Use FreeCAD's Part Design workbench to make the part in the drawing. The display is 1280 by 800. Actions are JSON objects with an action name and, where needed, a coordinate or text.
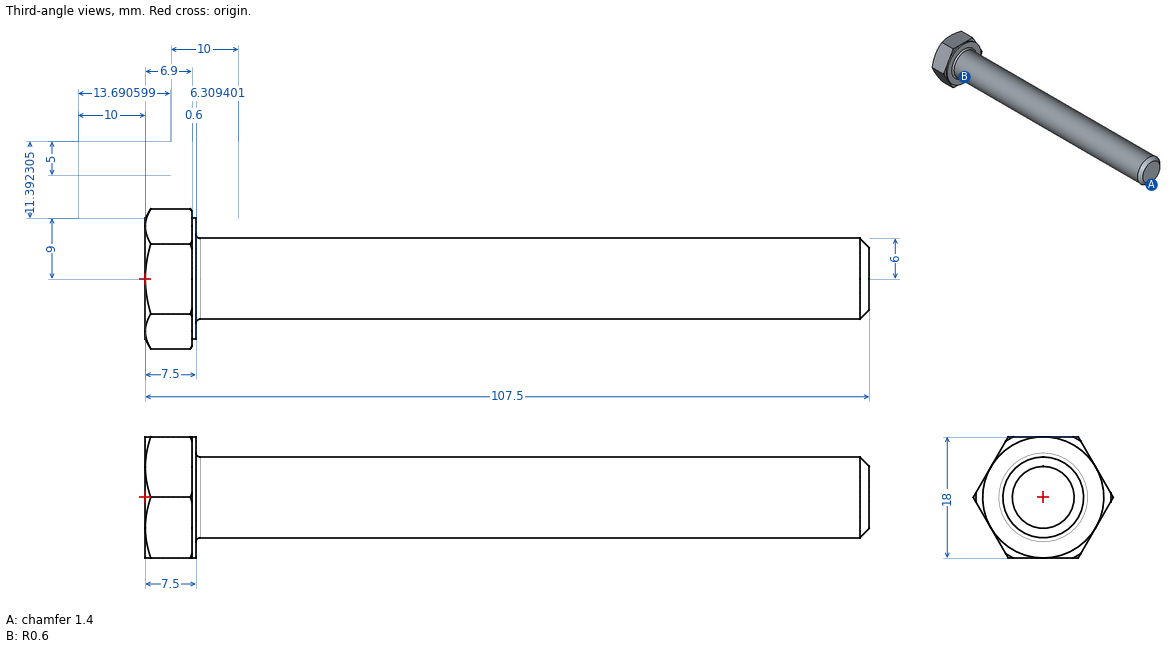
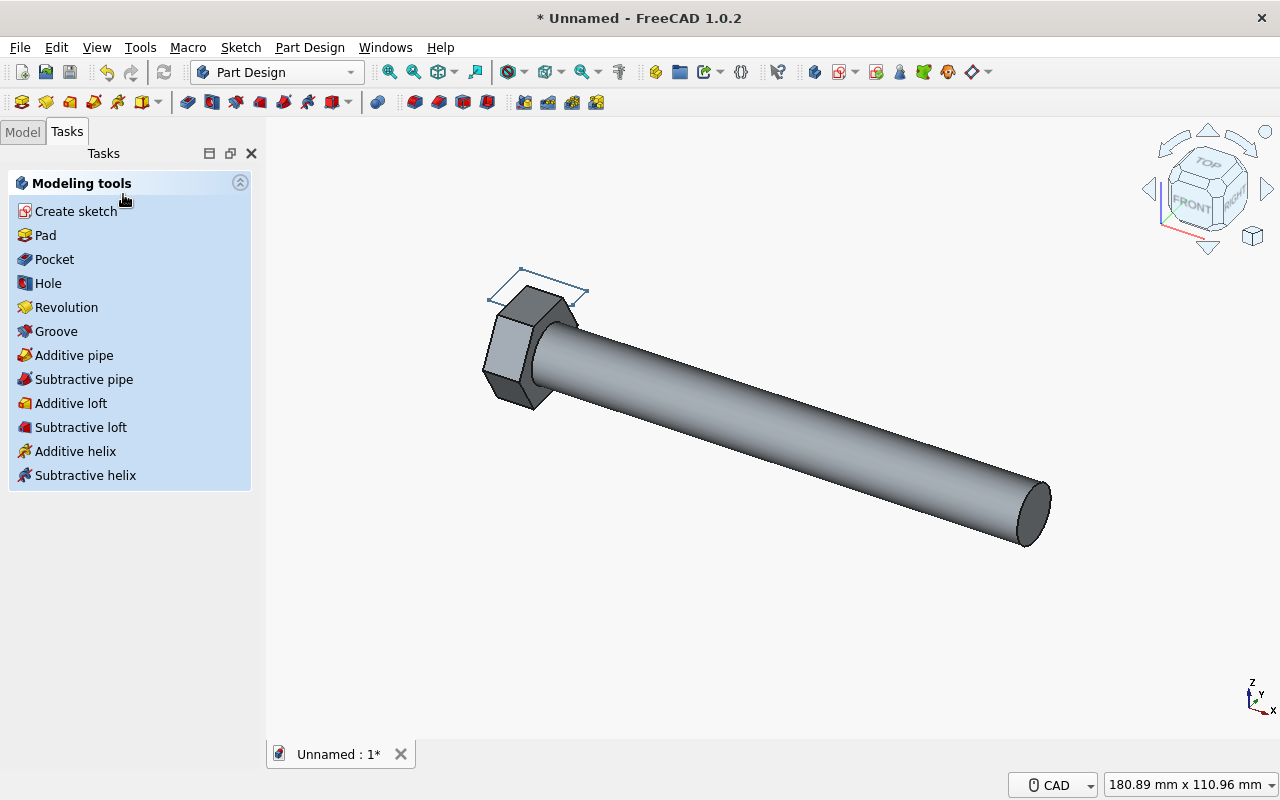
{"action": "left_click", "coordinate": [236, 102]}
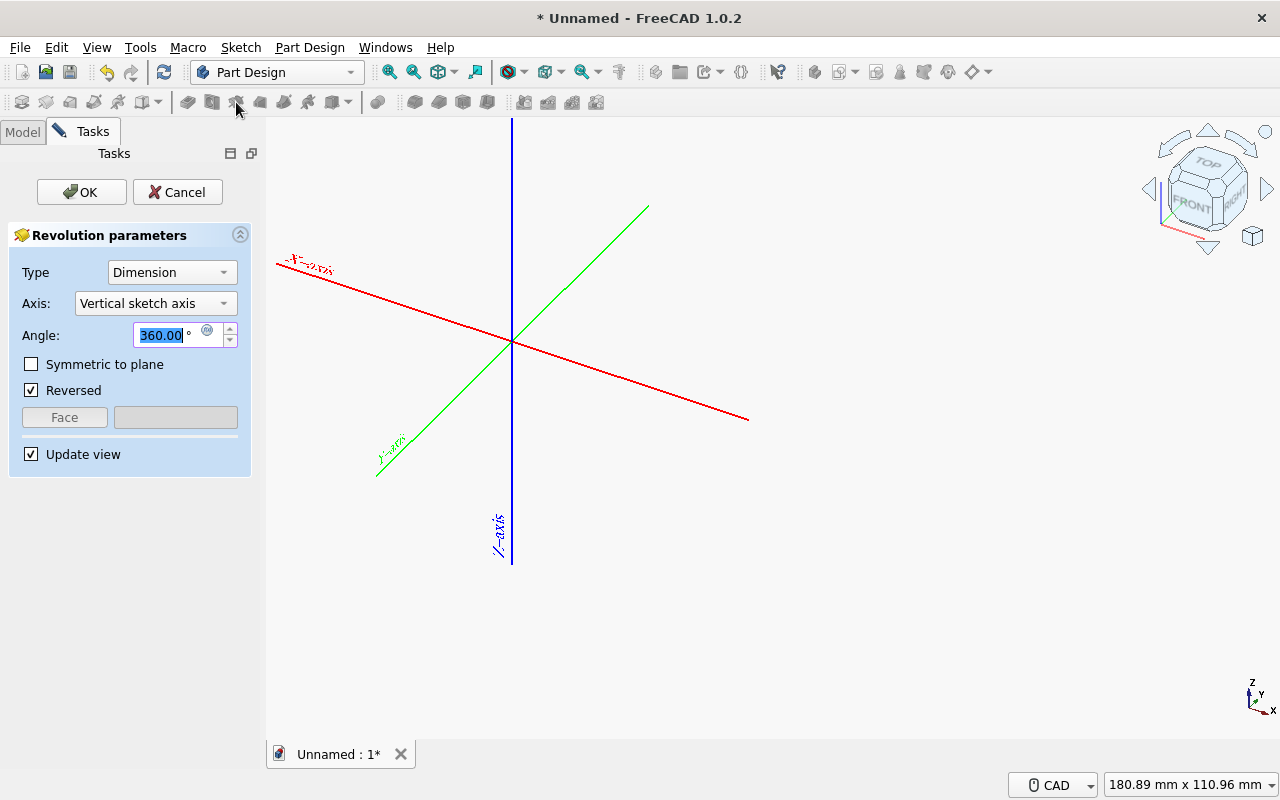
{"action": "left_click", "coordinate": [156, 304]}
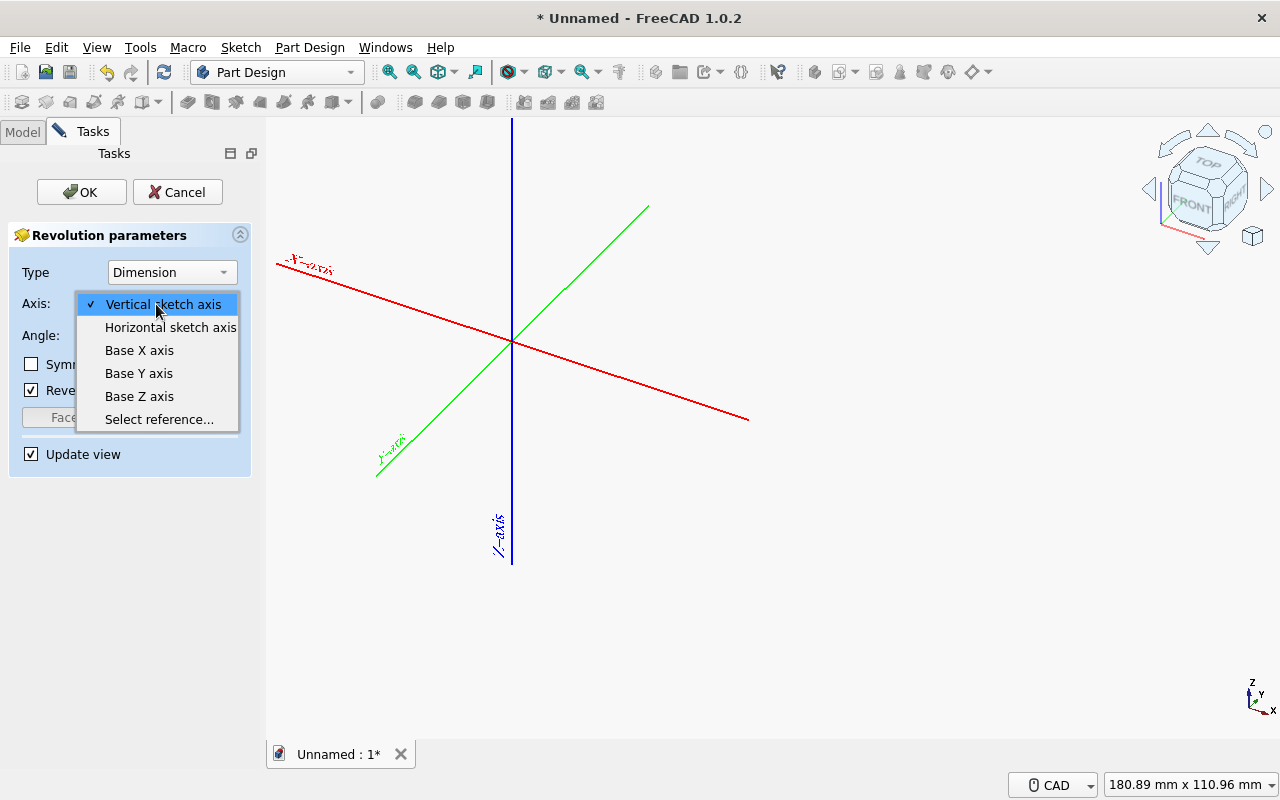
{"action": "left_click", "coordinate": [156, 328]}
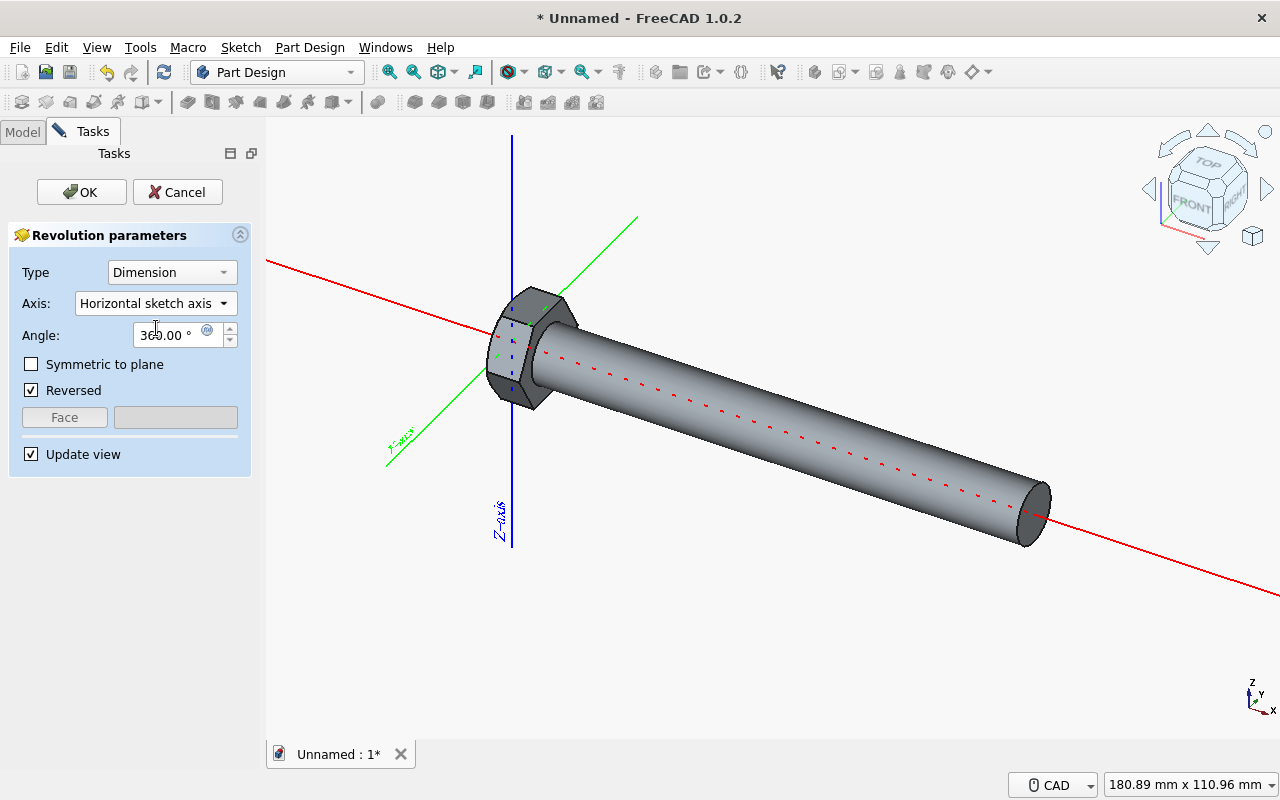
{"action": "left_click", "coordinate": [82, 192]}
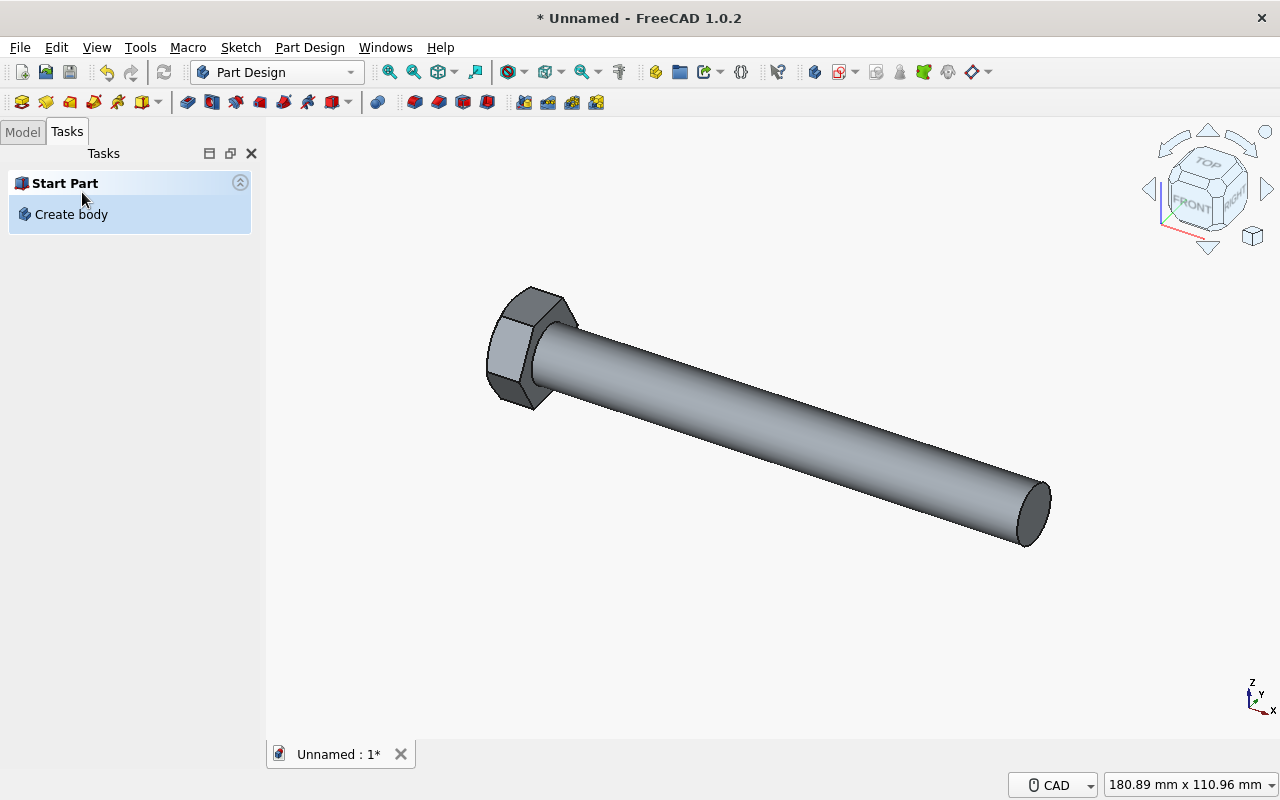
{"action": "left_click", "coordinate": [840, 72]}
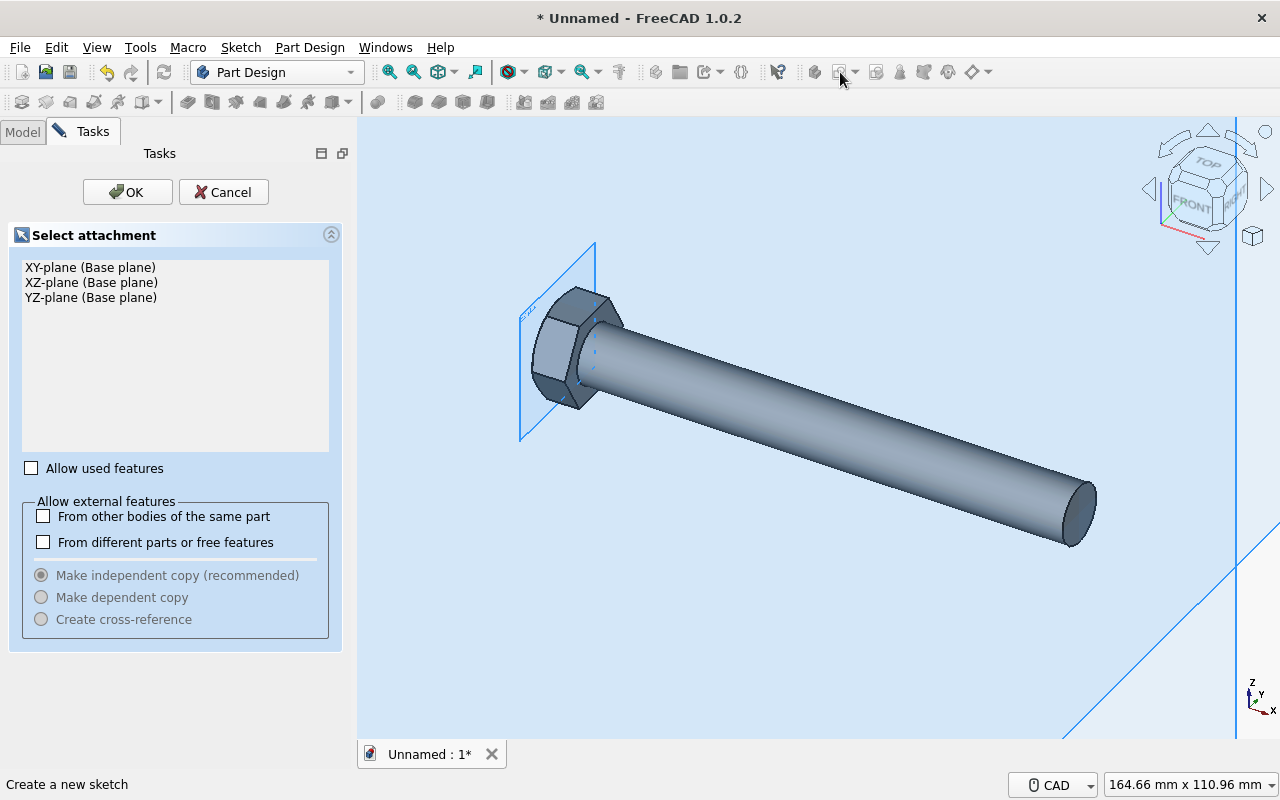
{"action": "left_click", "coordinate": [82, 268]}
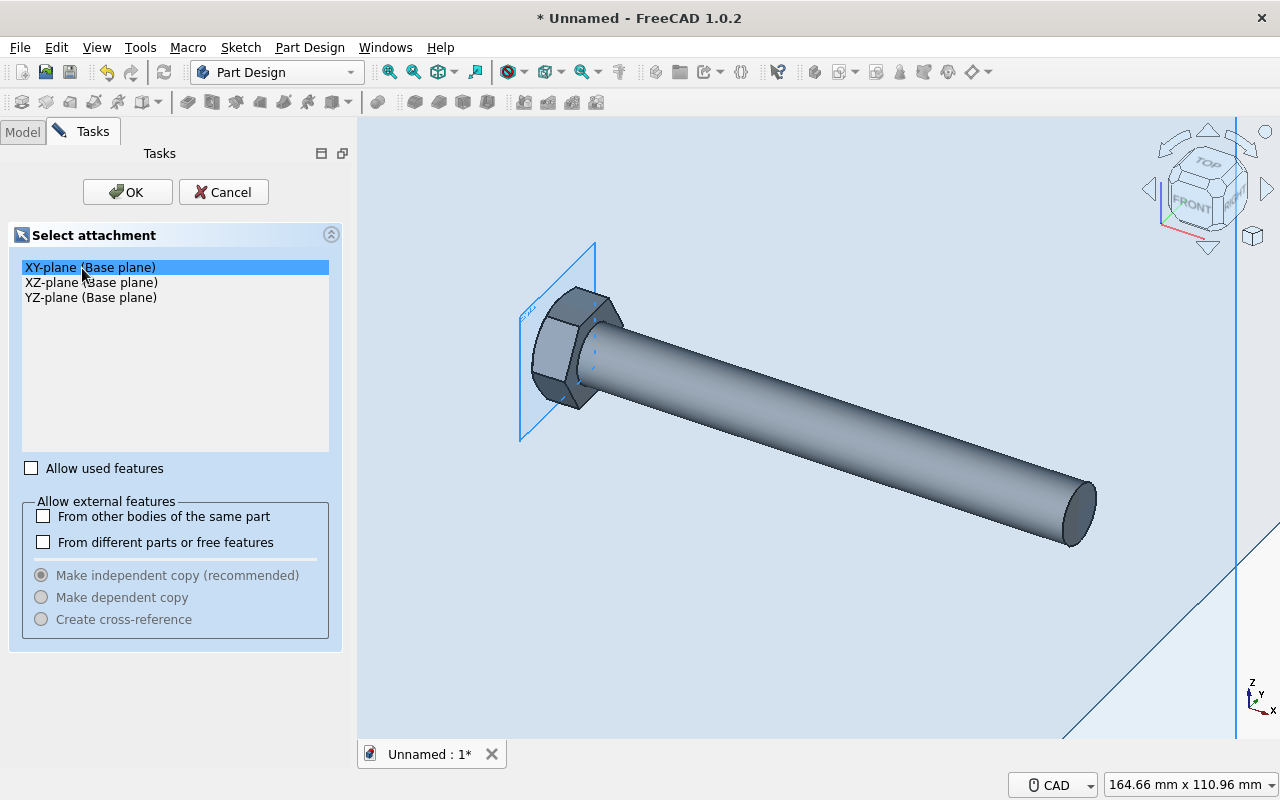
{"action": "left_click", "coordinate": [128, 192]}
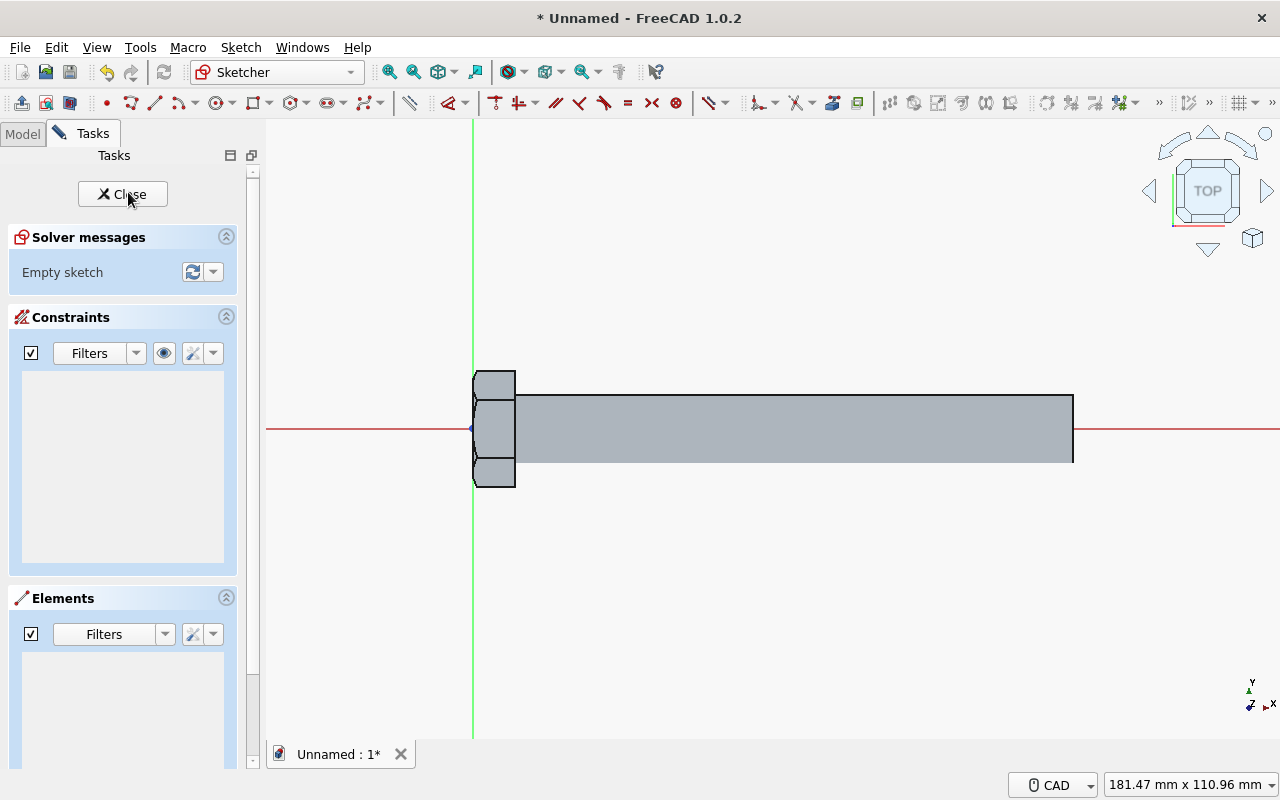
{"action": "key", "text": "q s"}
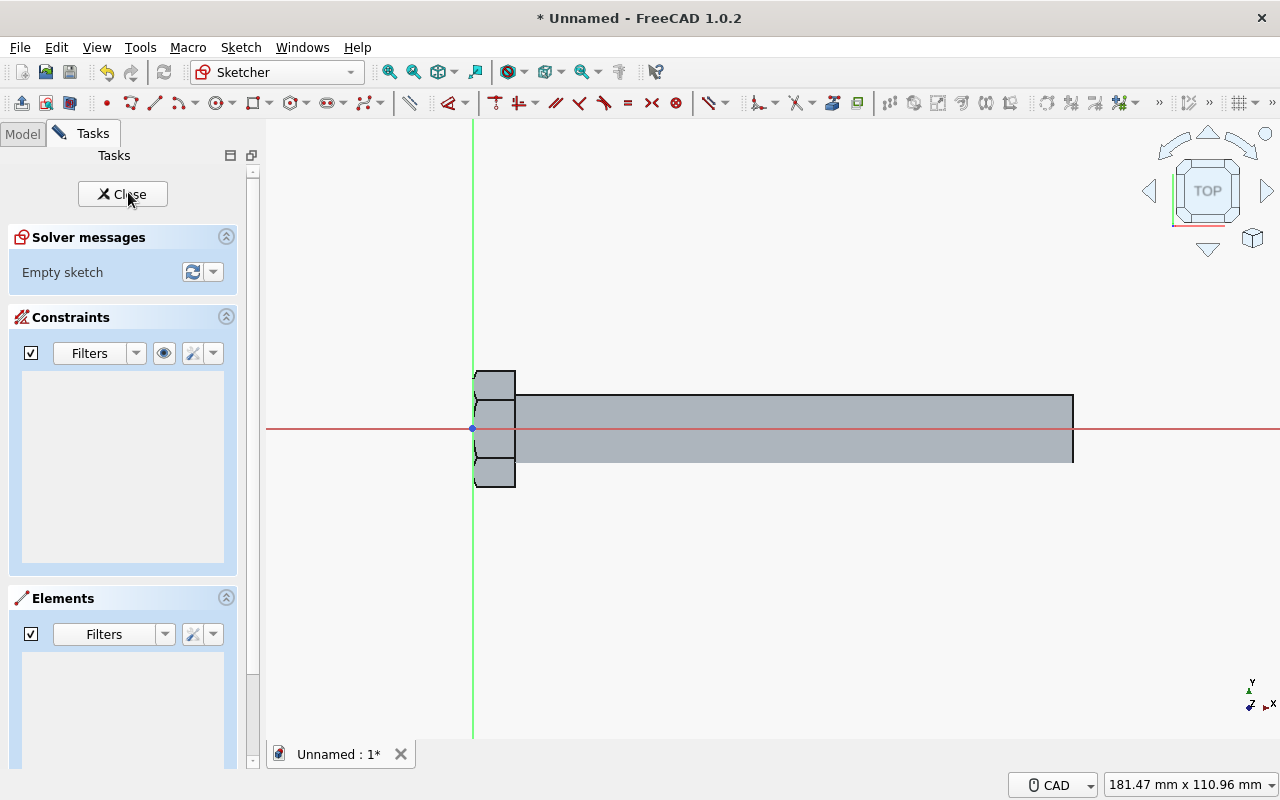
{"action": "scroll", "coordinate": [428, 347], "scroll_direction": "up", "scroll_amount": 6}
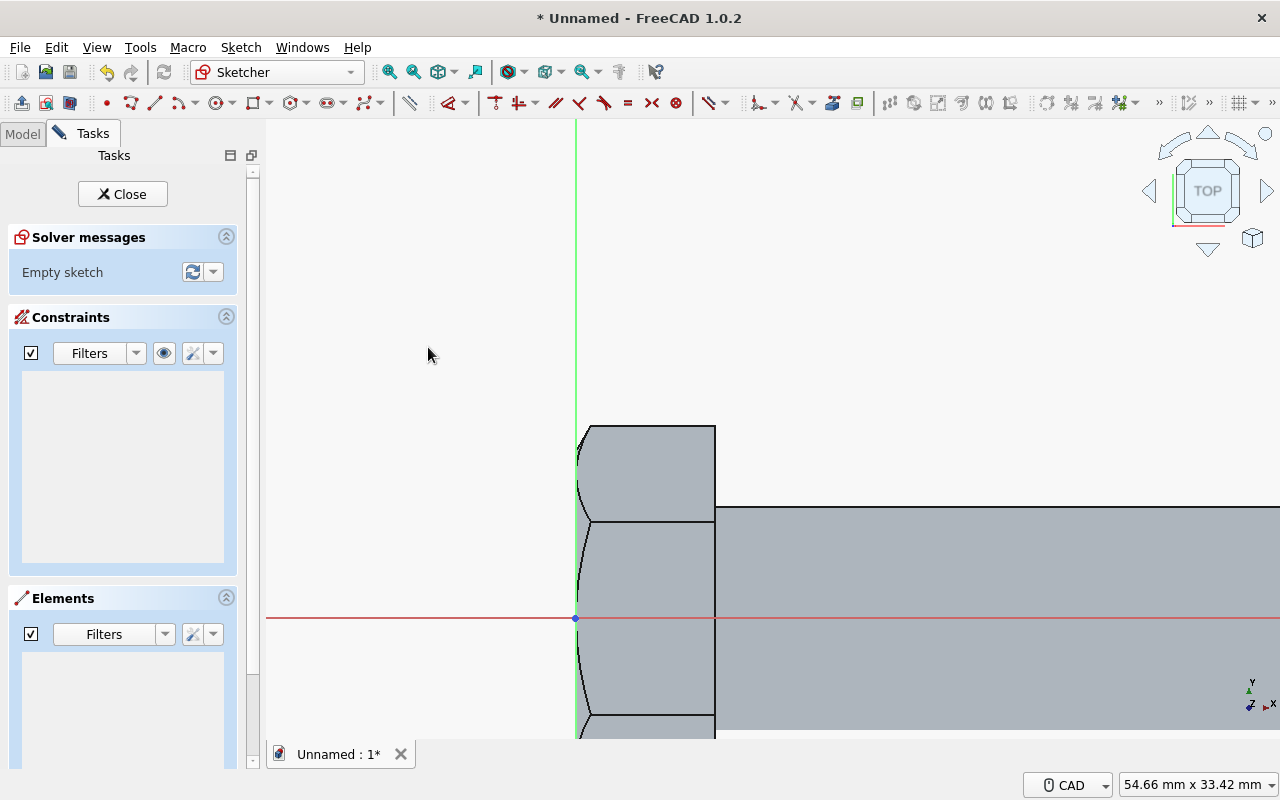
{"action": "key", "text": "g m"}